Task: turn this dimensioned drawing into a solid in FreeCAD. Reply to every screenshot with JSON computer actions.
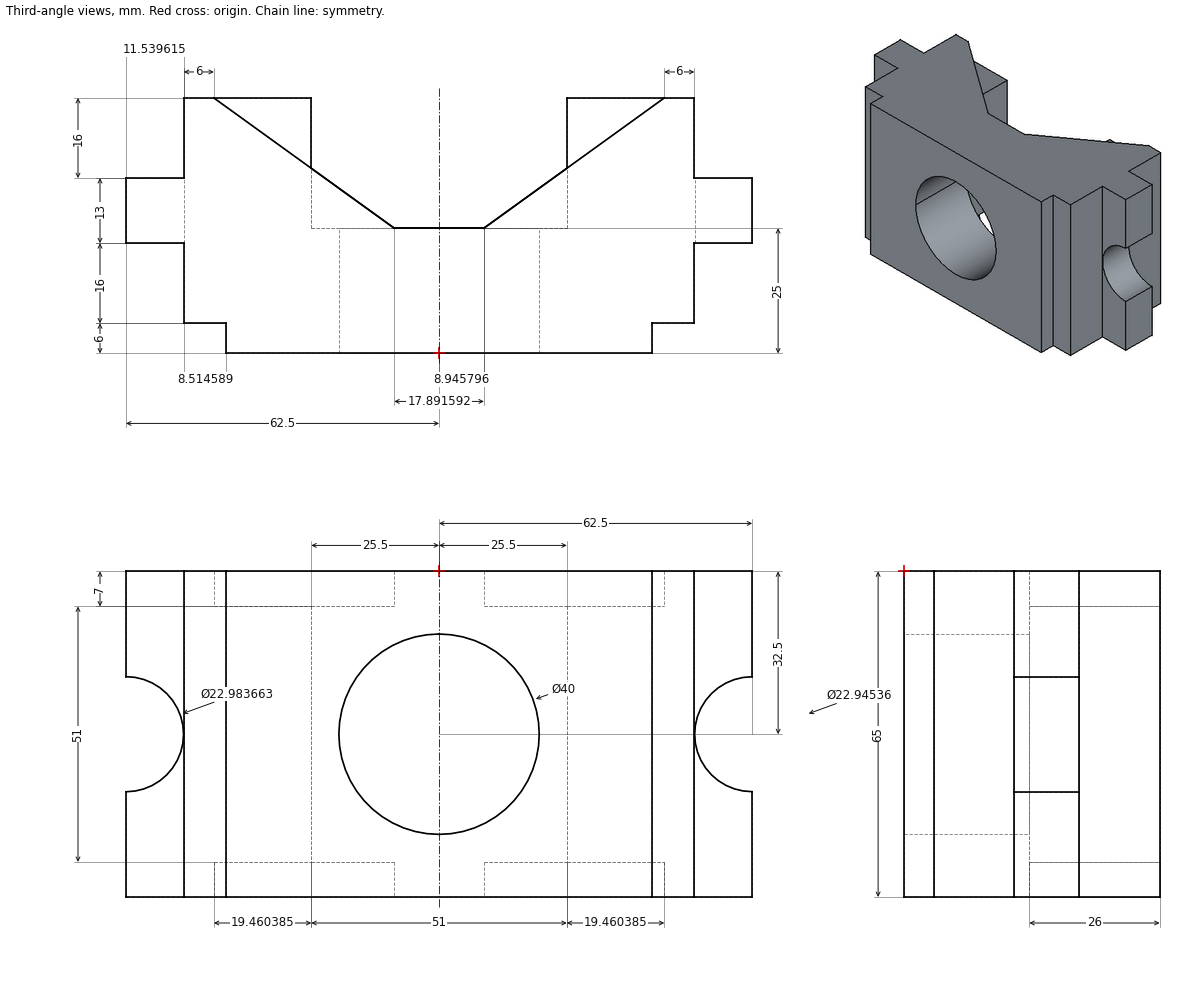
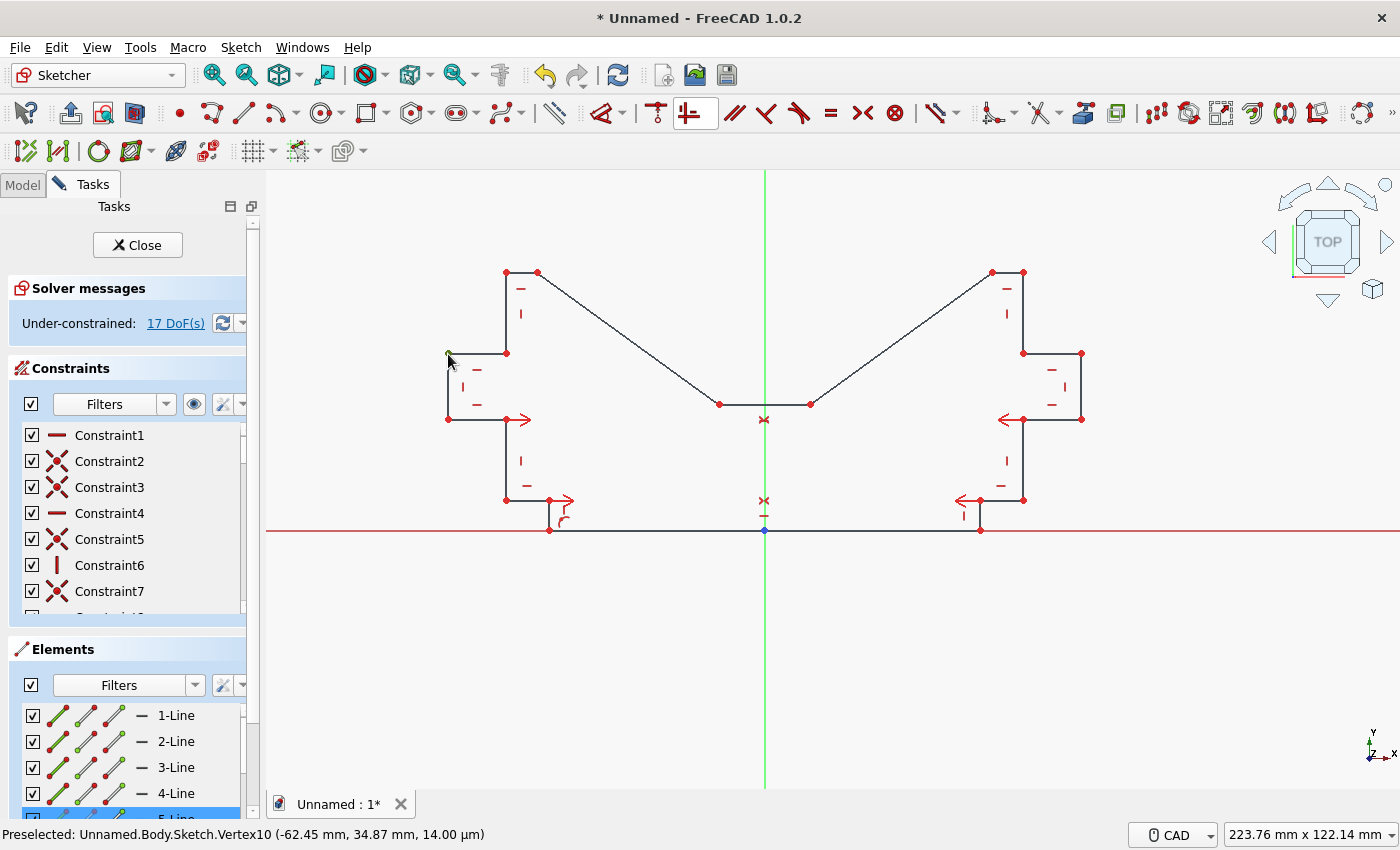
{"action": "left_click", "coordinate": [1081, 354]}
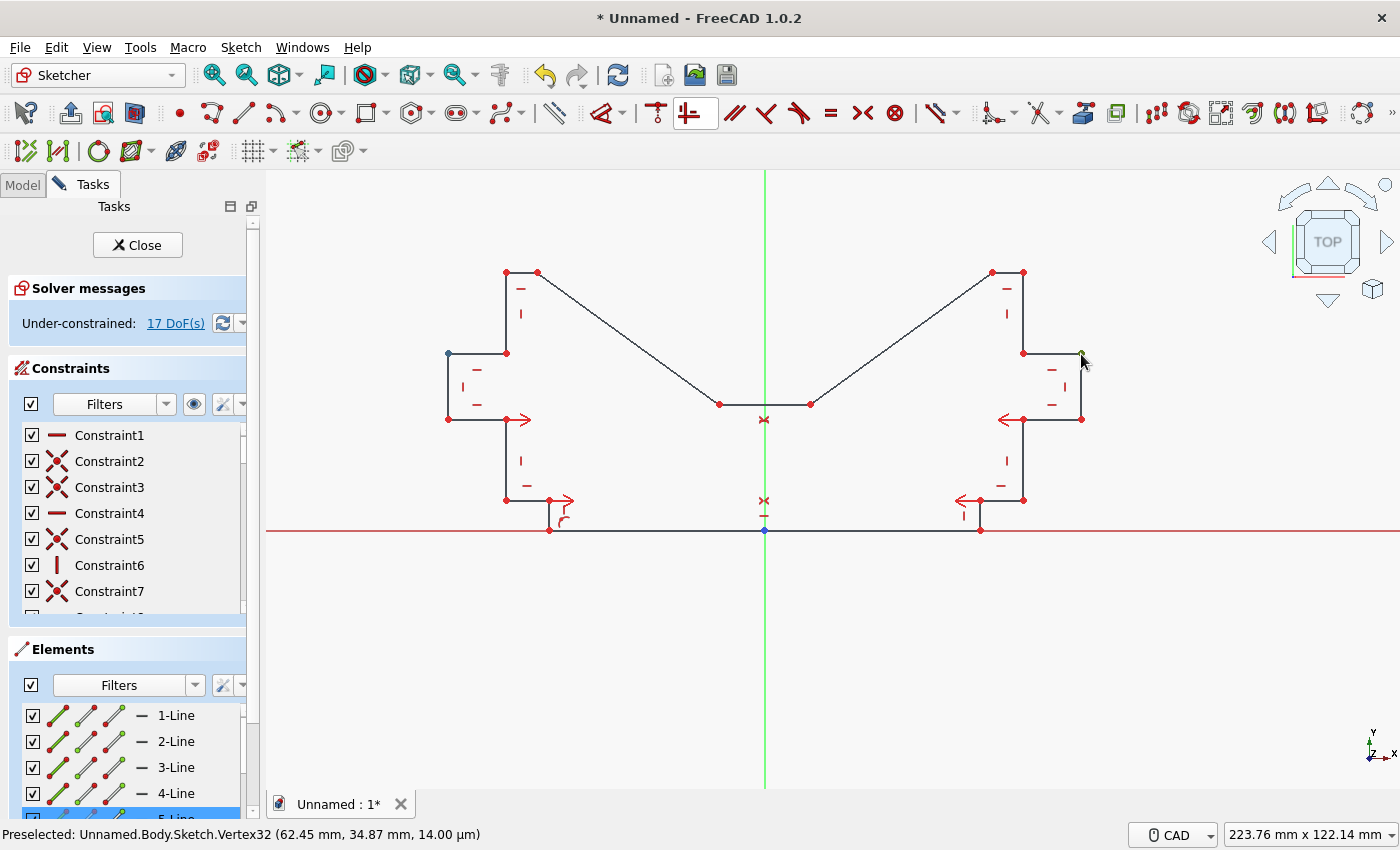
{"action": "left_click", "coordinate": [765, 721]}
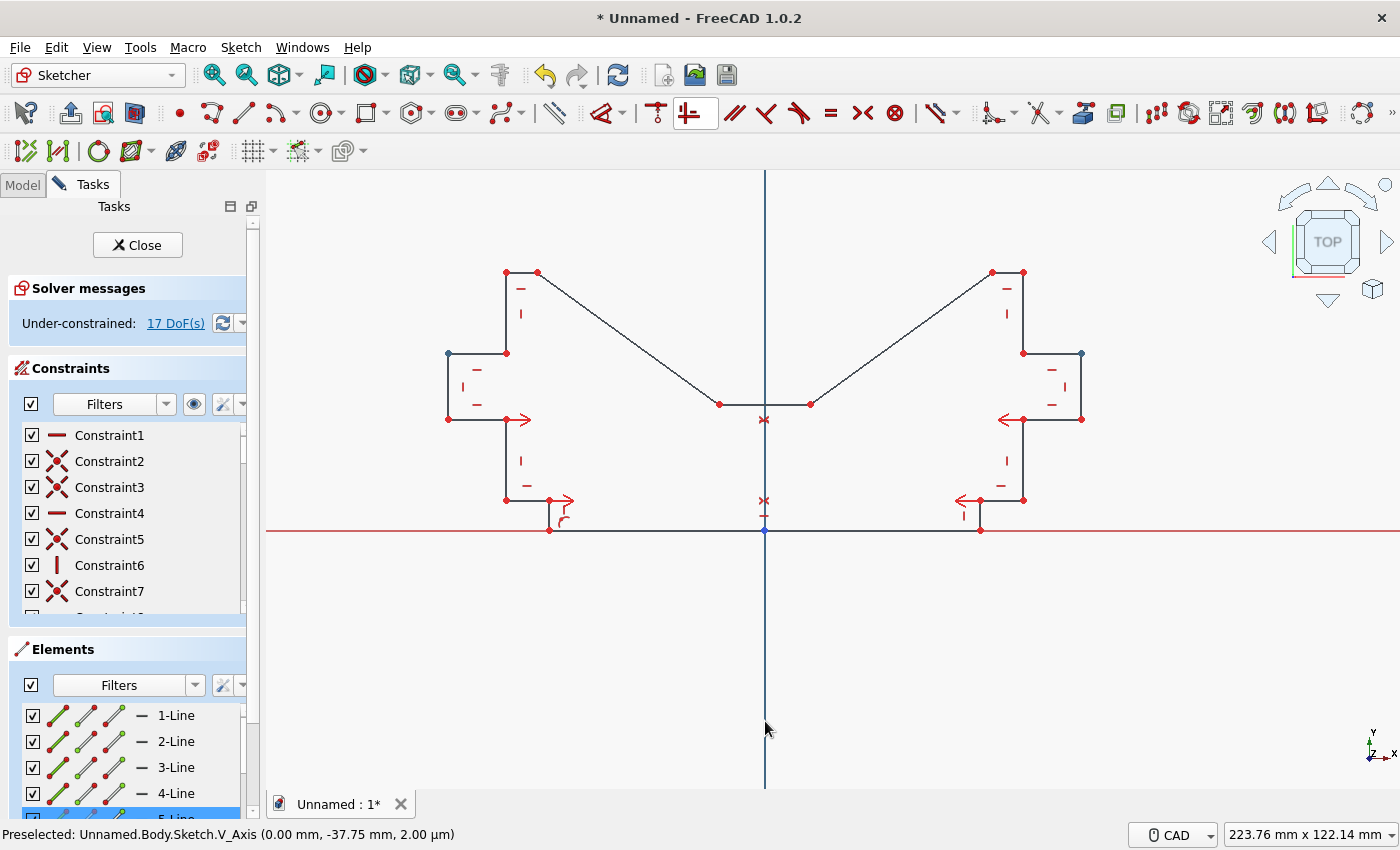
{"action": "left_click", "coordinate": [864, 114]}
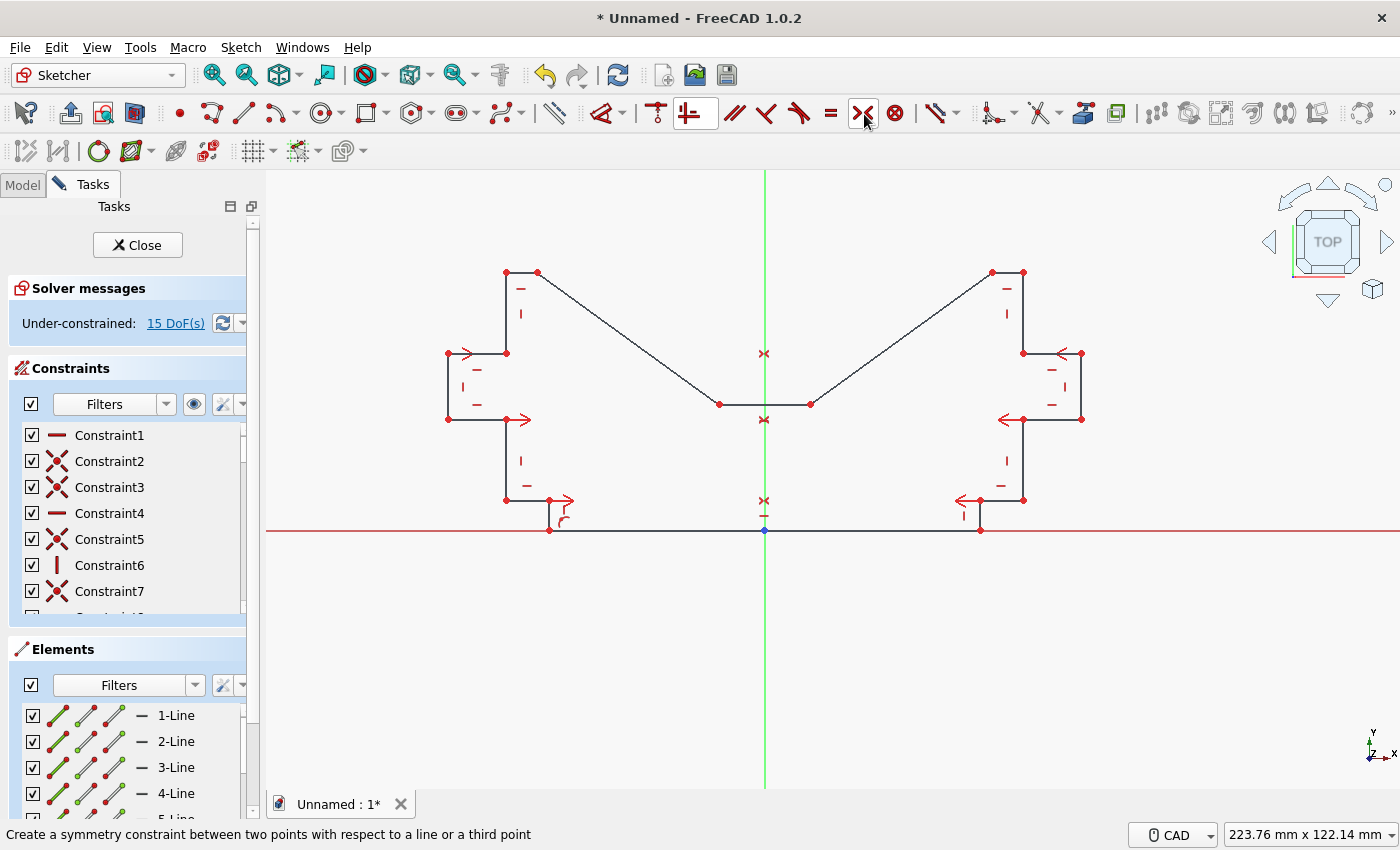
{"action": "left_click", "coordinate": [506, 273]}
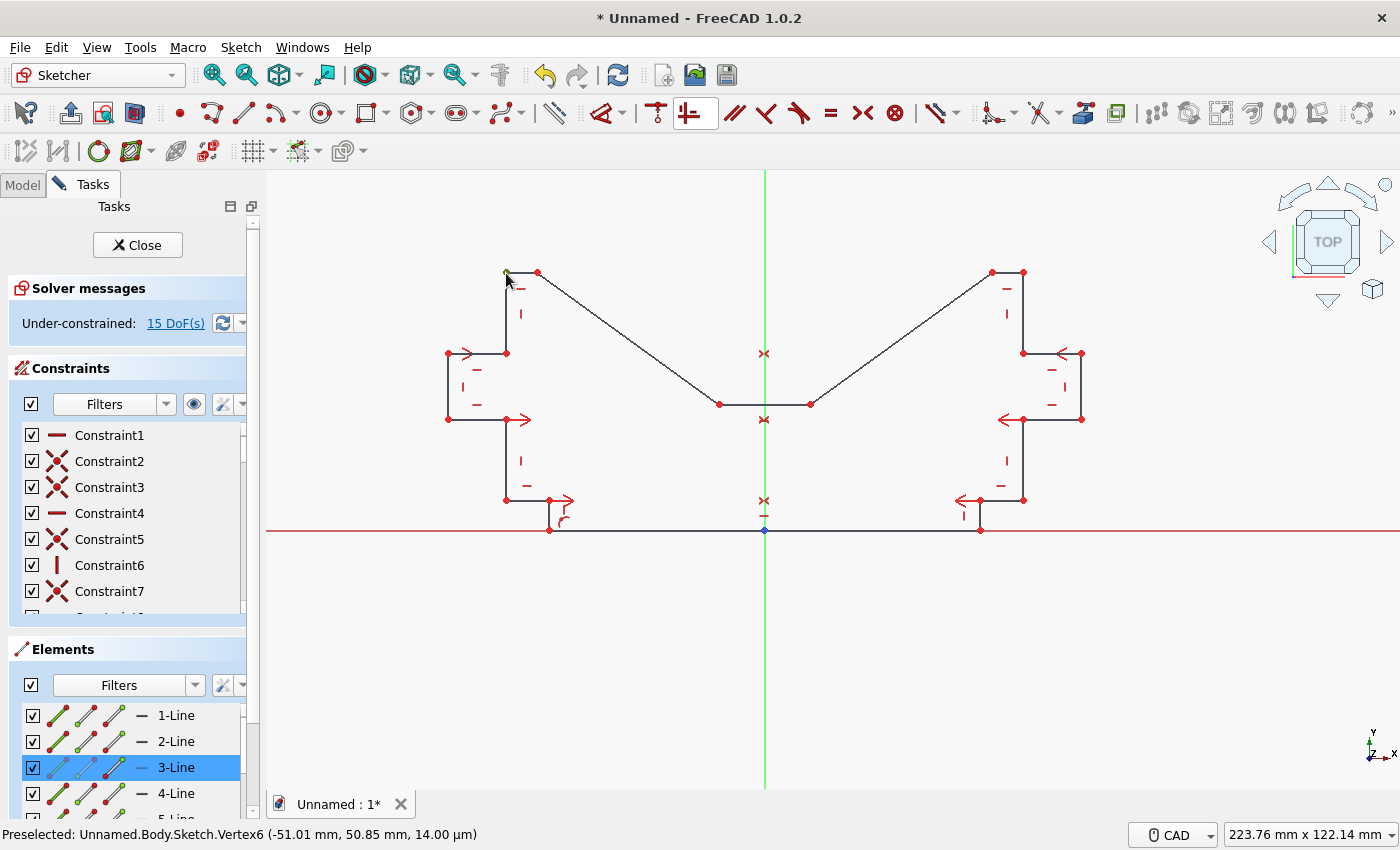
{"action": "left_click", "coordinate": [1023, 273]}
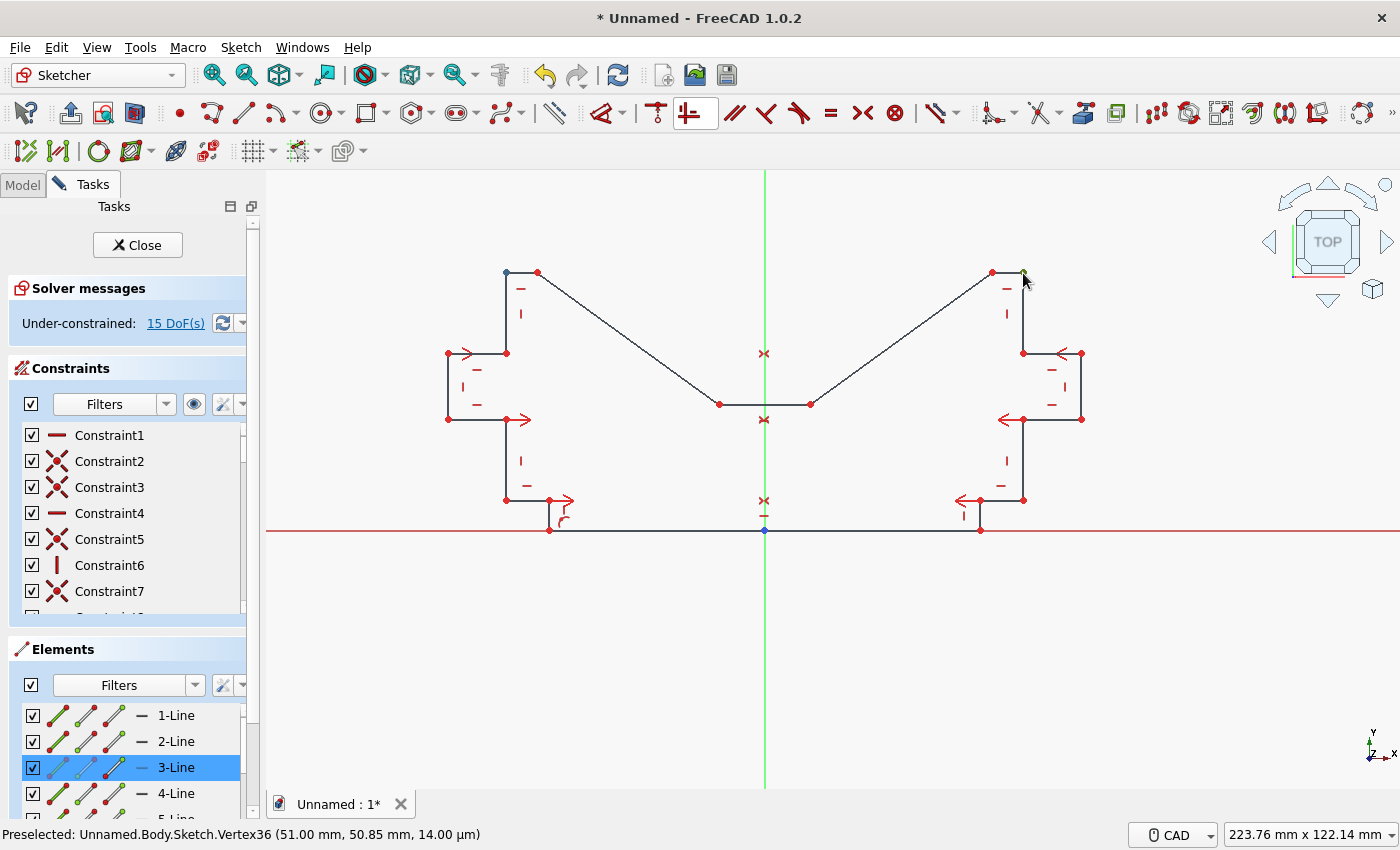
{"action": "left_click", "coordinate": [765, 721]}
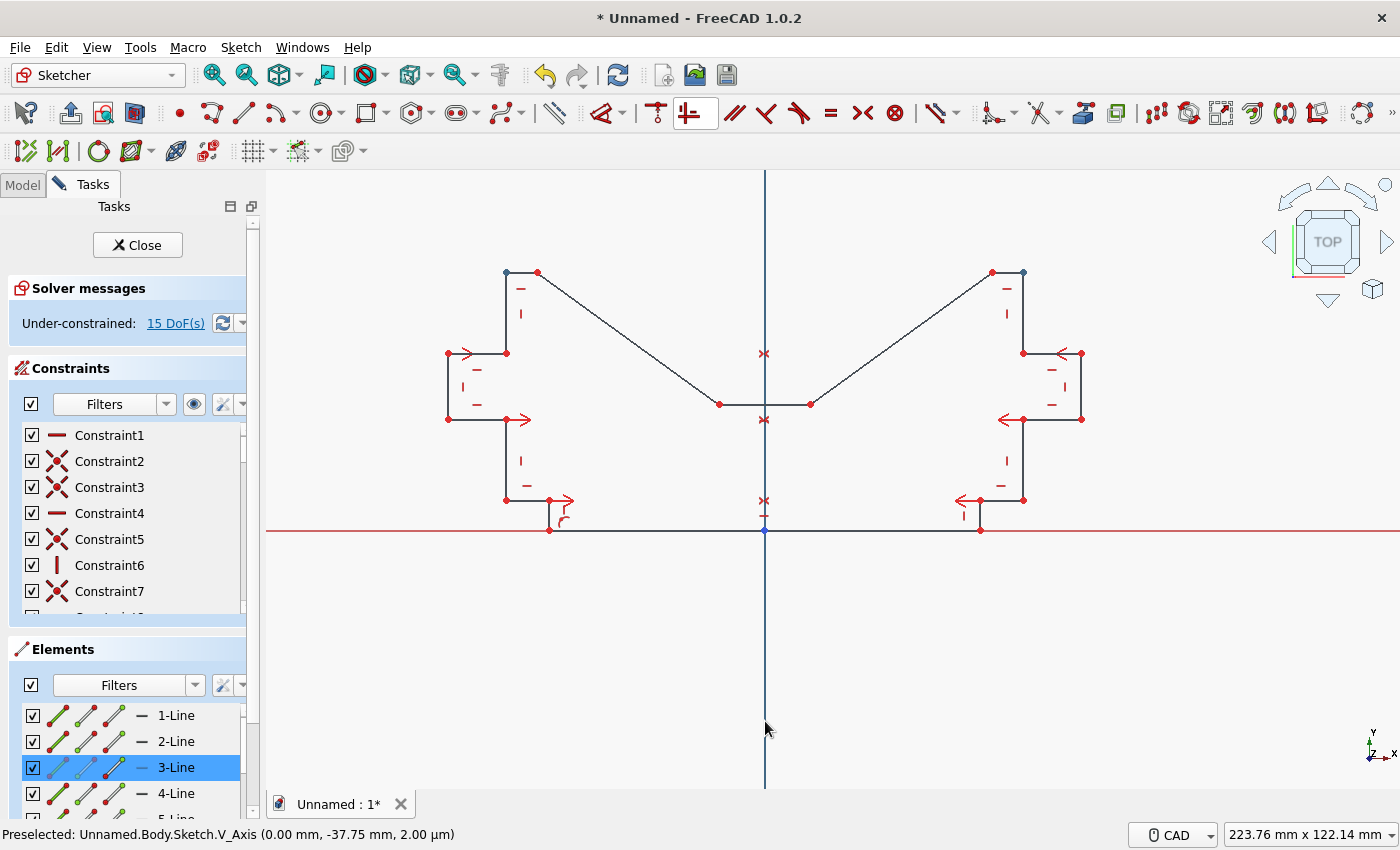
{"action": "left_click", "coordinate": [864, 114]}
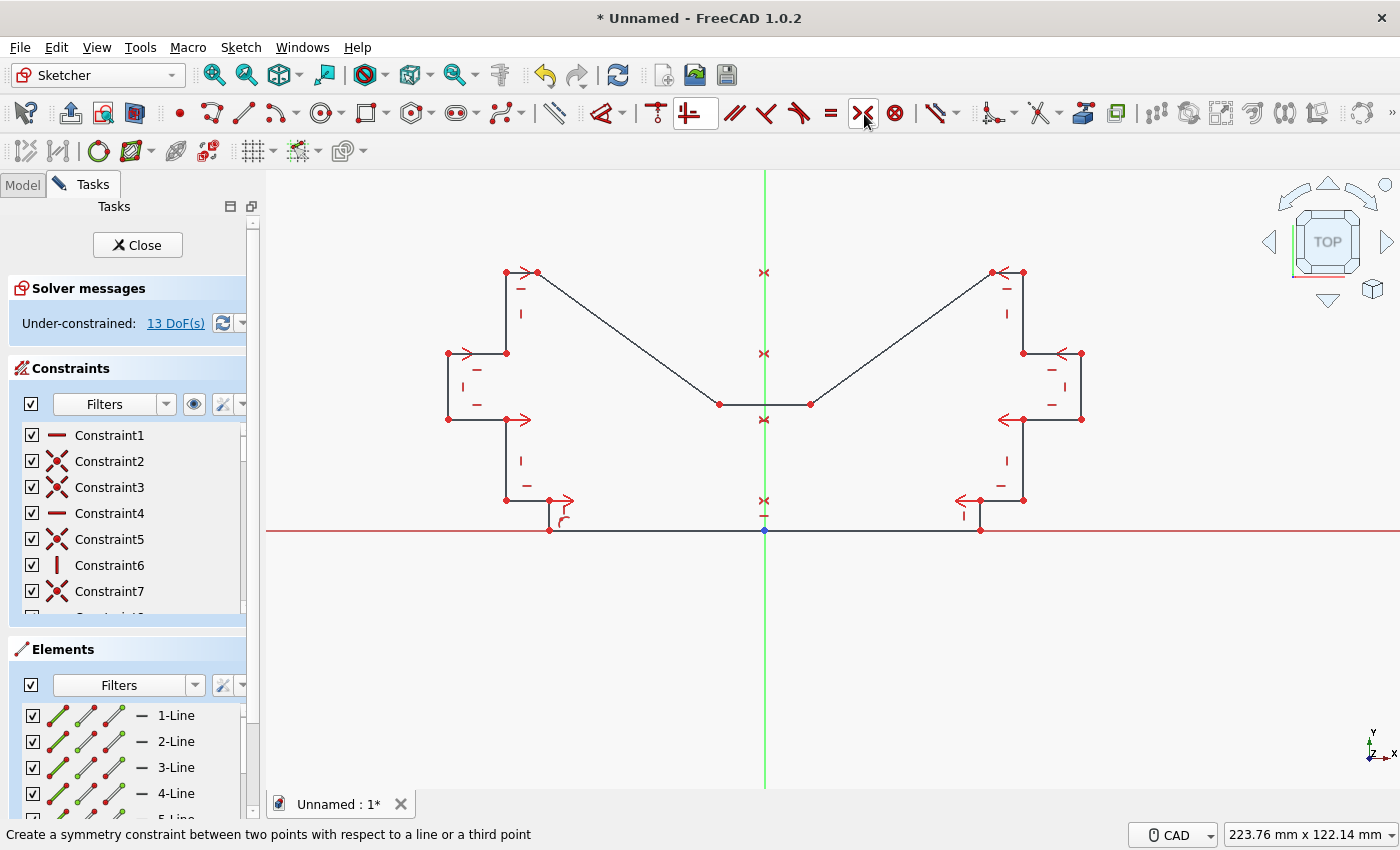
{"action": "left_click", "coordinate": [602, 114]}